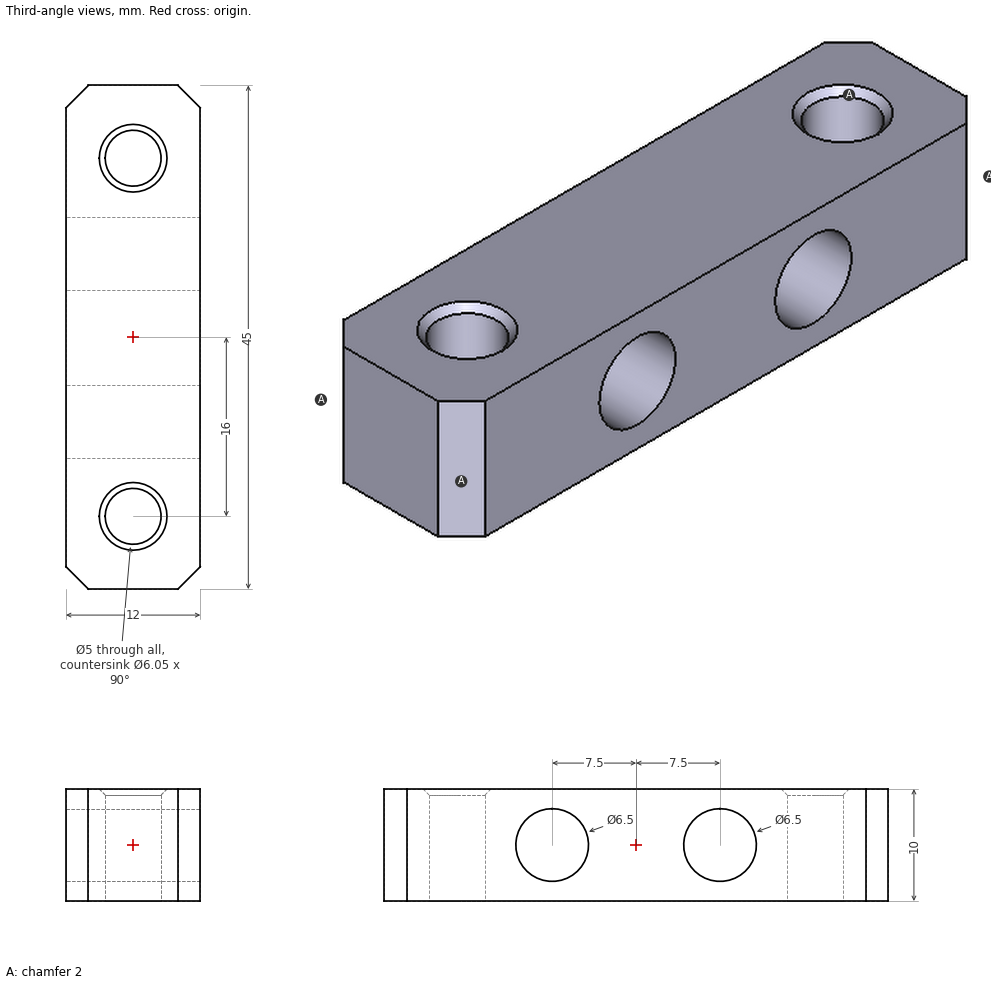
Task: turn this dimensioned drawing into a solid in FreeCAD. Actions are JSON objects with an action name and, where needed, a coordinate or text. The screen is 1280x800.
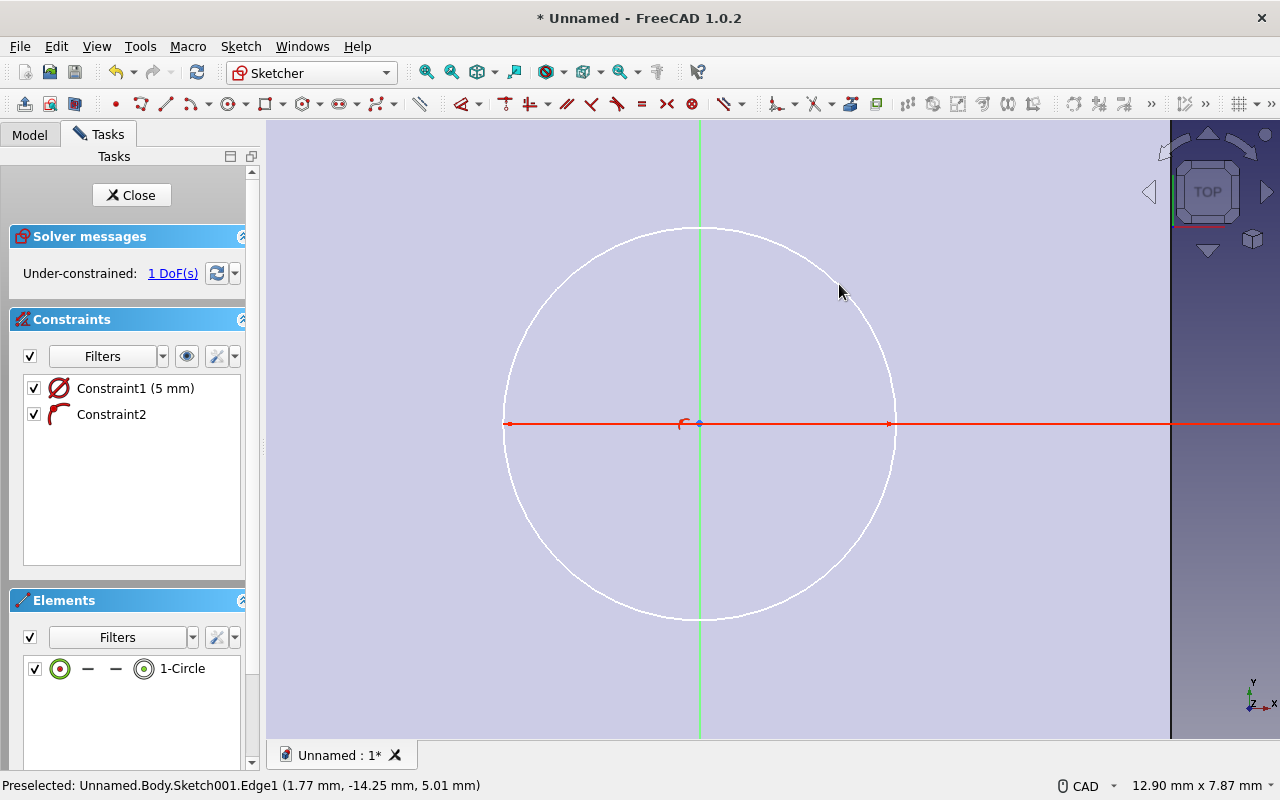
{"action": "left_click", "coordinate": [460, 104]}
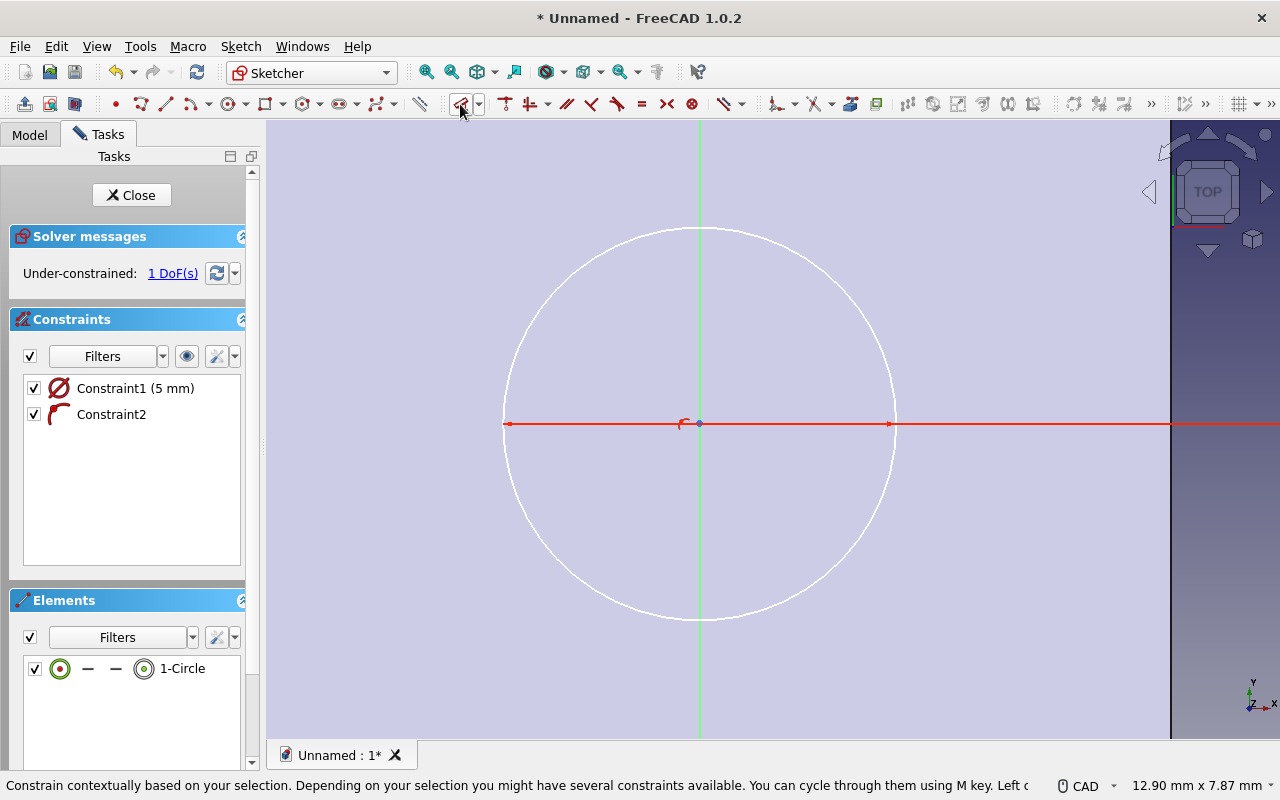
{"action": "left_click", "coordinate": [700, 424]}
{"action": "left_click", "coordinate": [734, 286]}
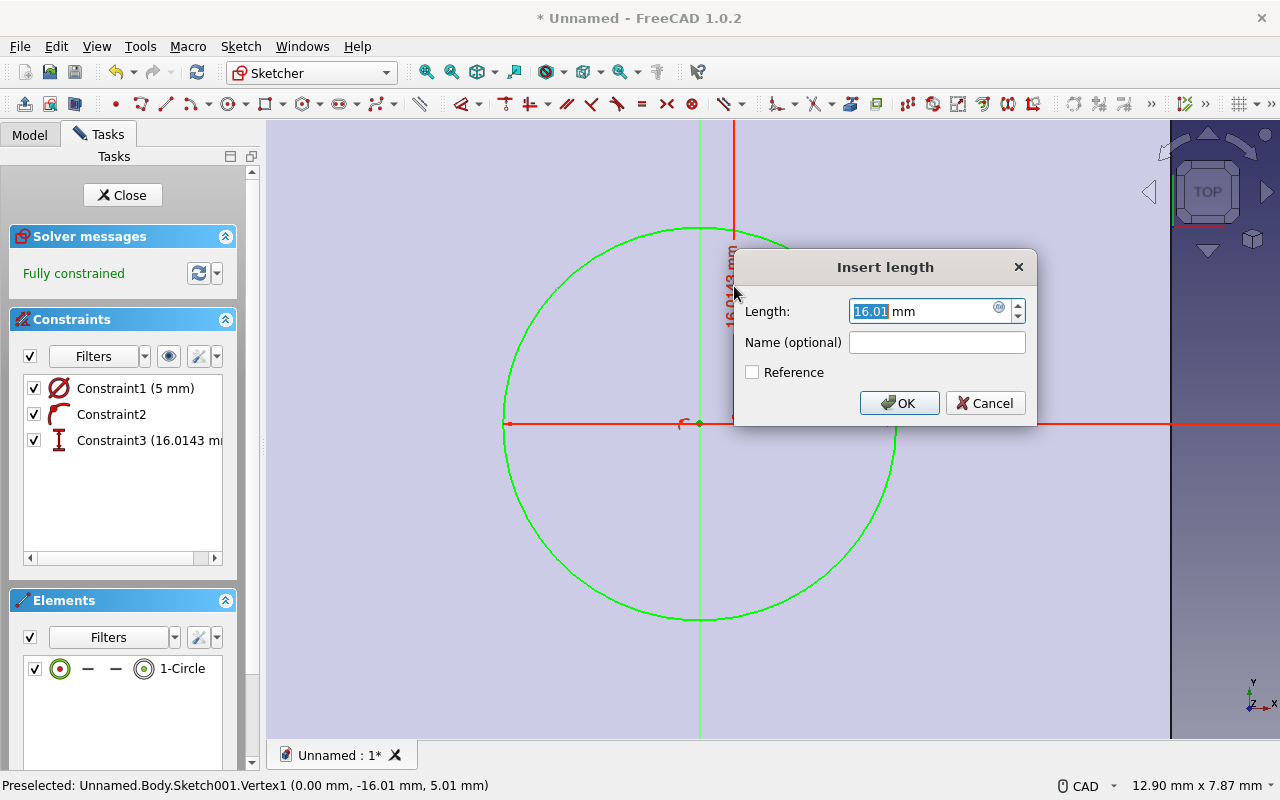
{"action": "type", "text": "16"}
{"action": "key", "text": "Return"}
{"action": "key", "text": "Escape"}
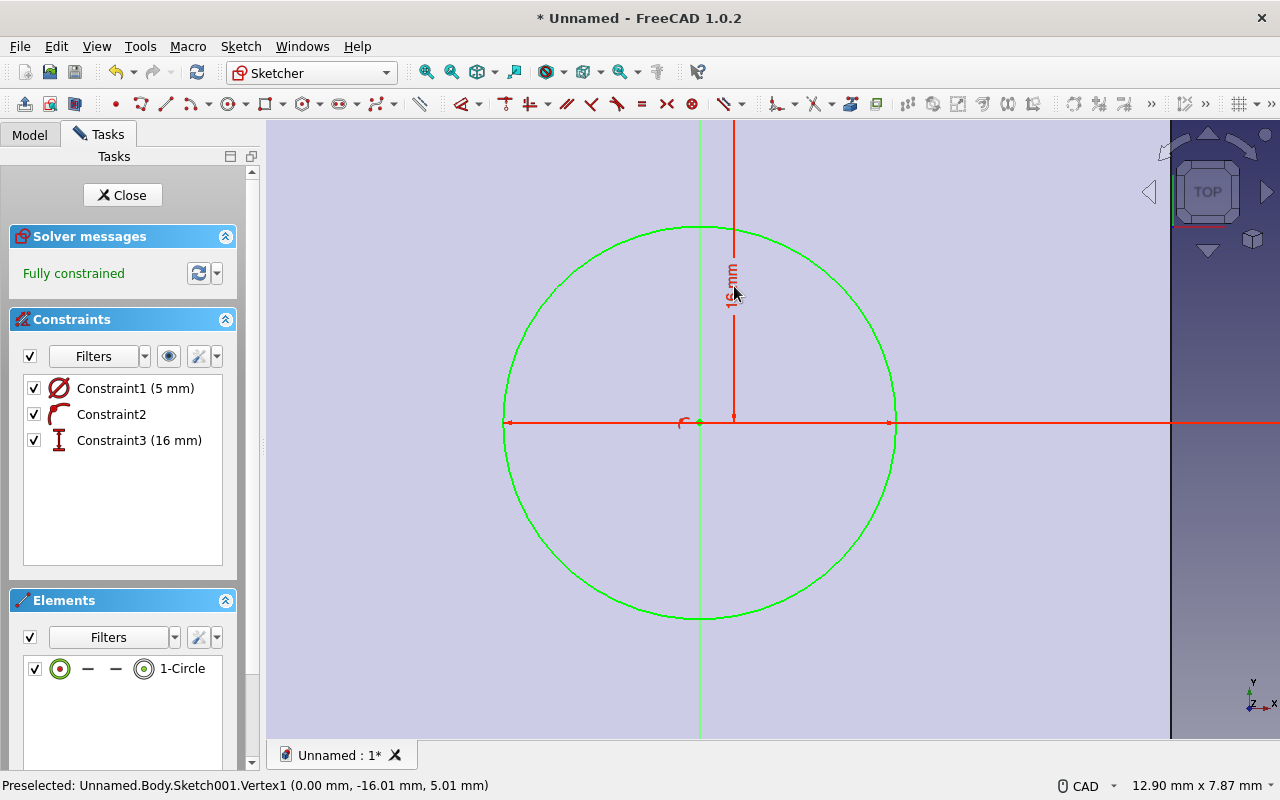
{"action": "left_click", "coordinate": [123, 195]}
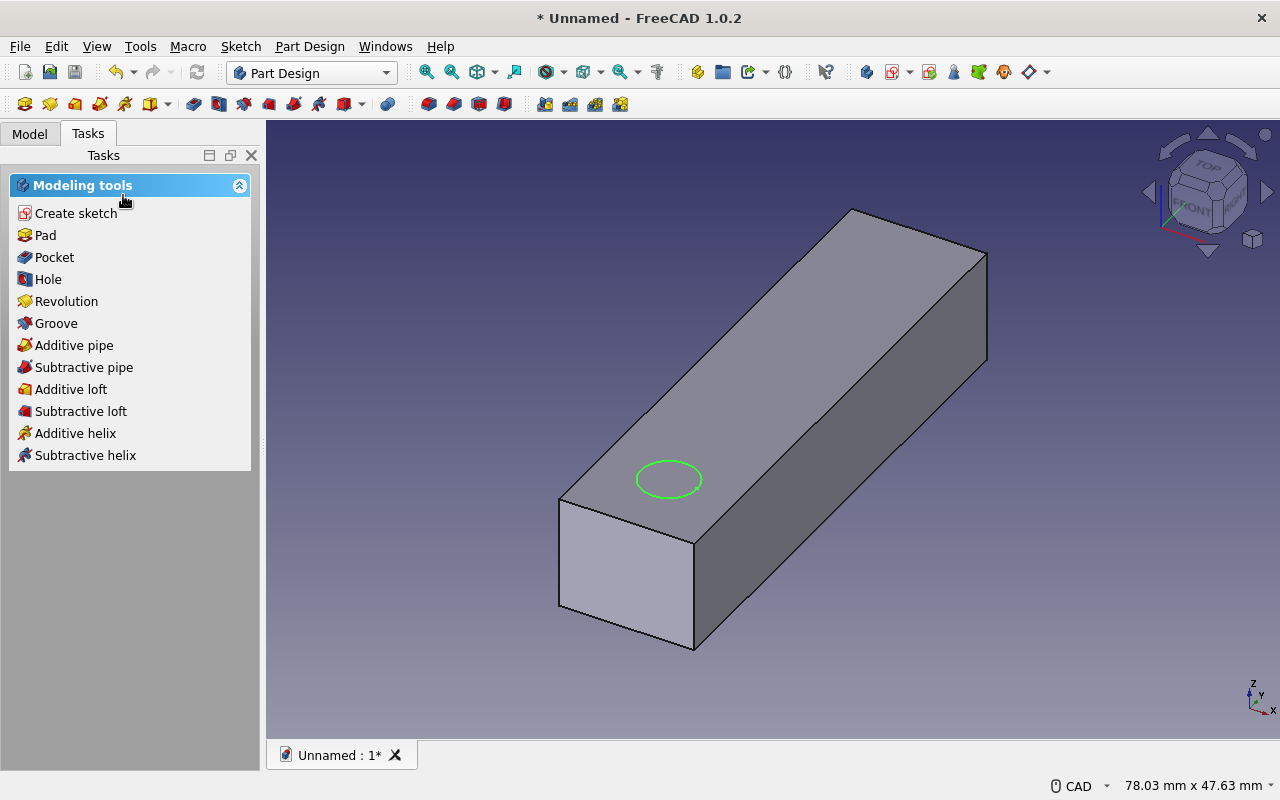
{"action": "left_click", "coordinate": [219, 104]}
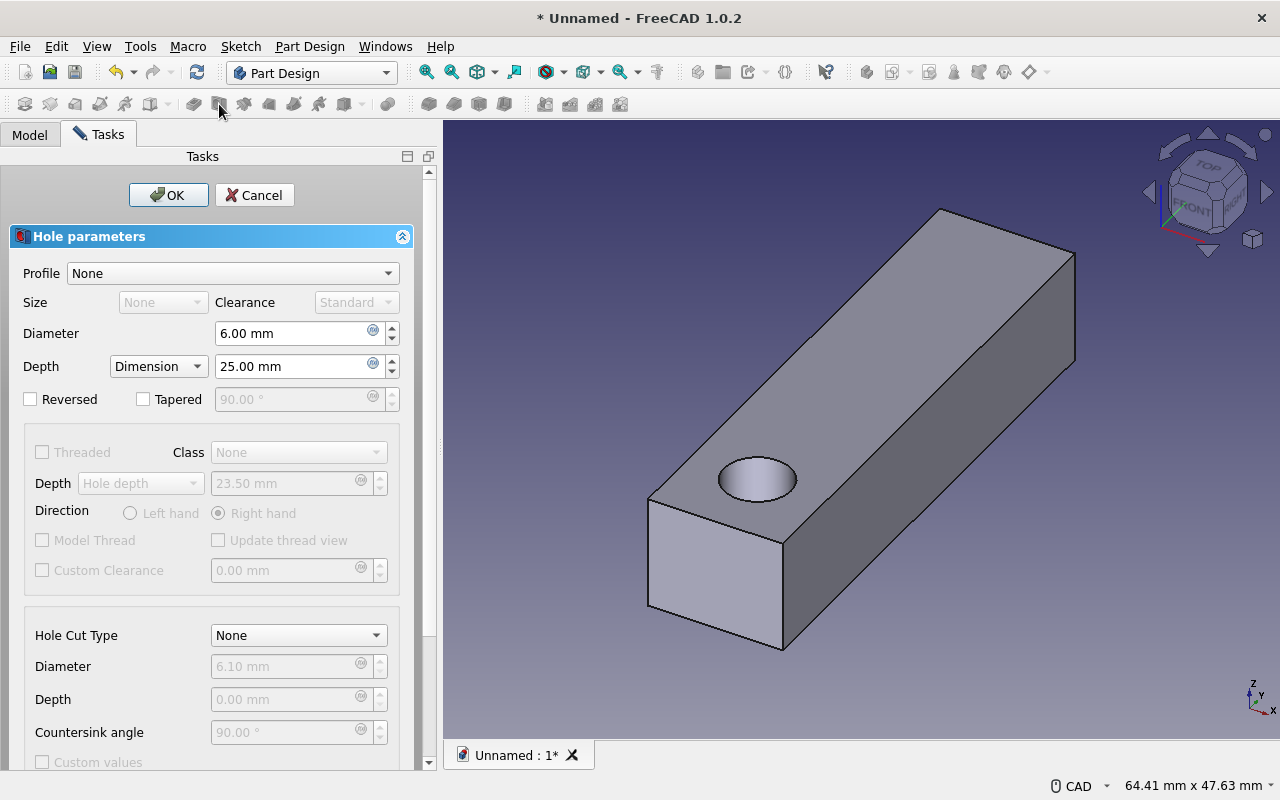
{"action": "triple_click", "coordinate": [300, 334]}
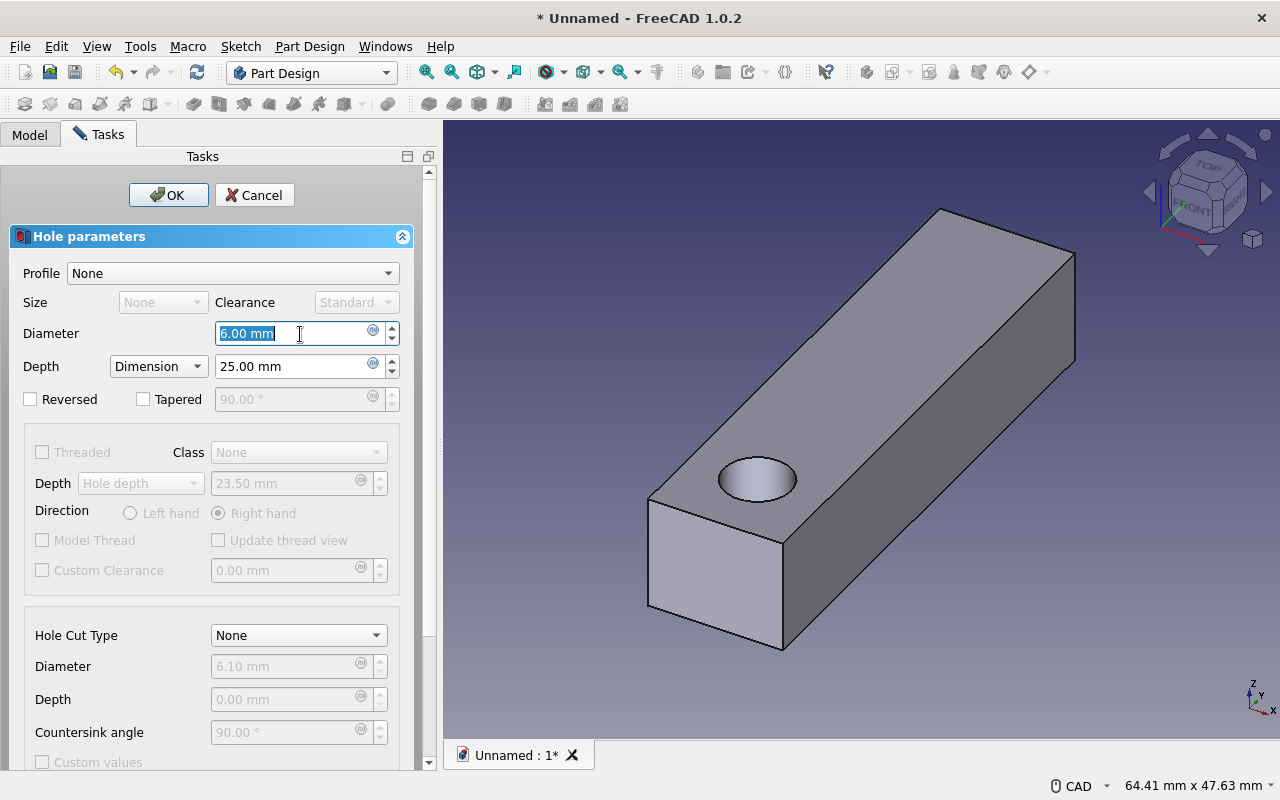
{"action": "type", "text": "5"}
{"action": "key", "text": "Tab"}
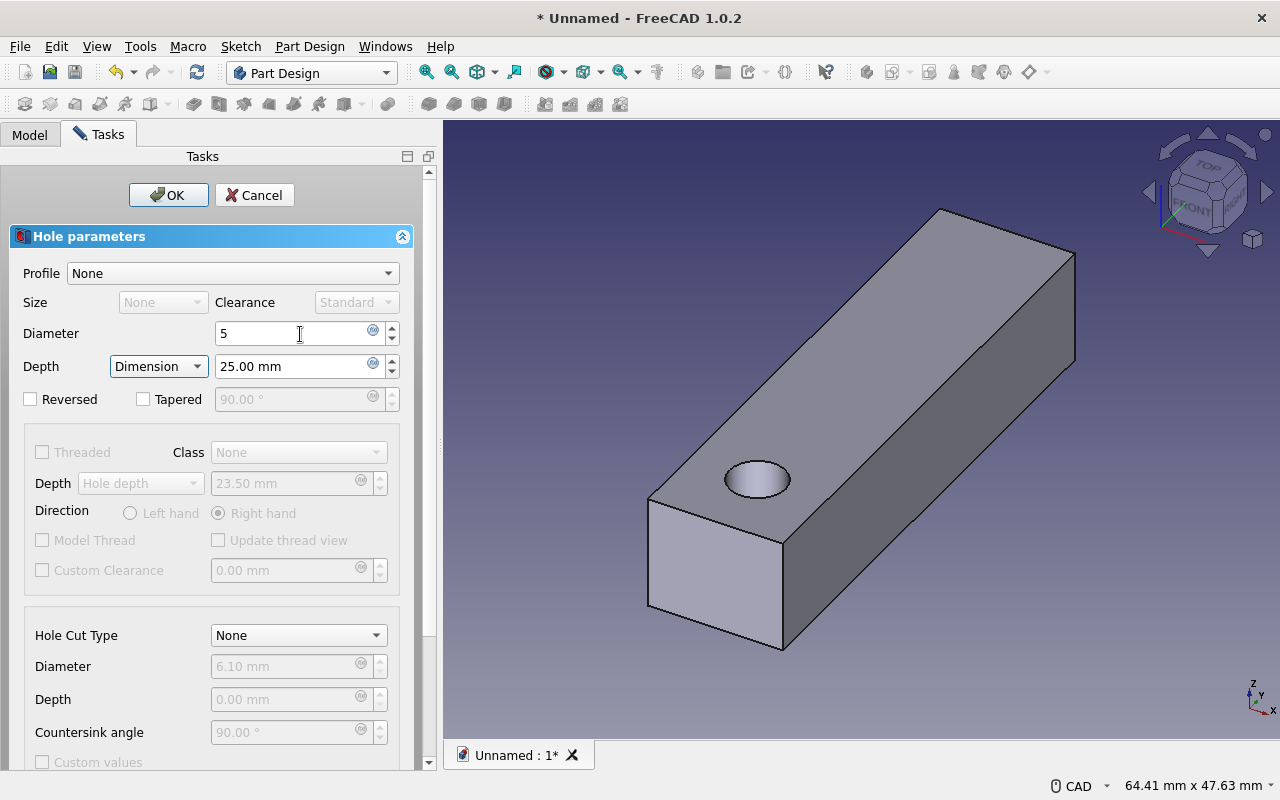
{"action": "left_click", "coordinate": [160, 366]}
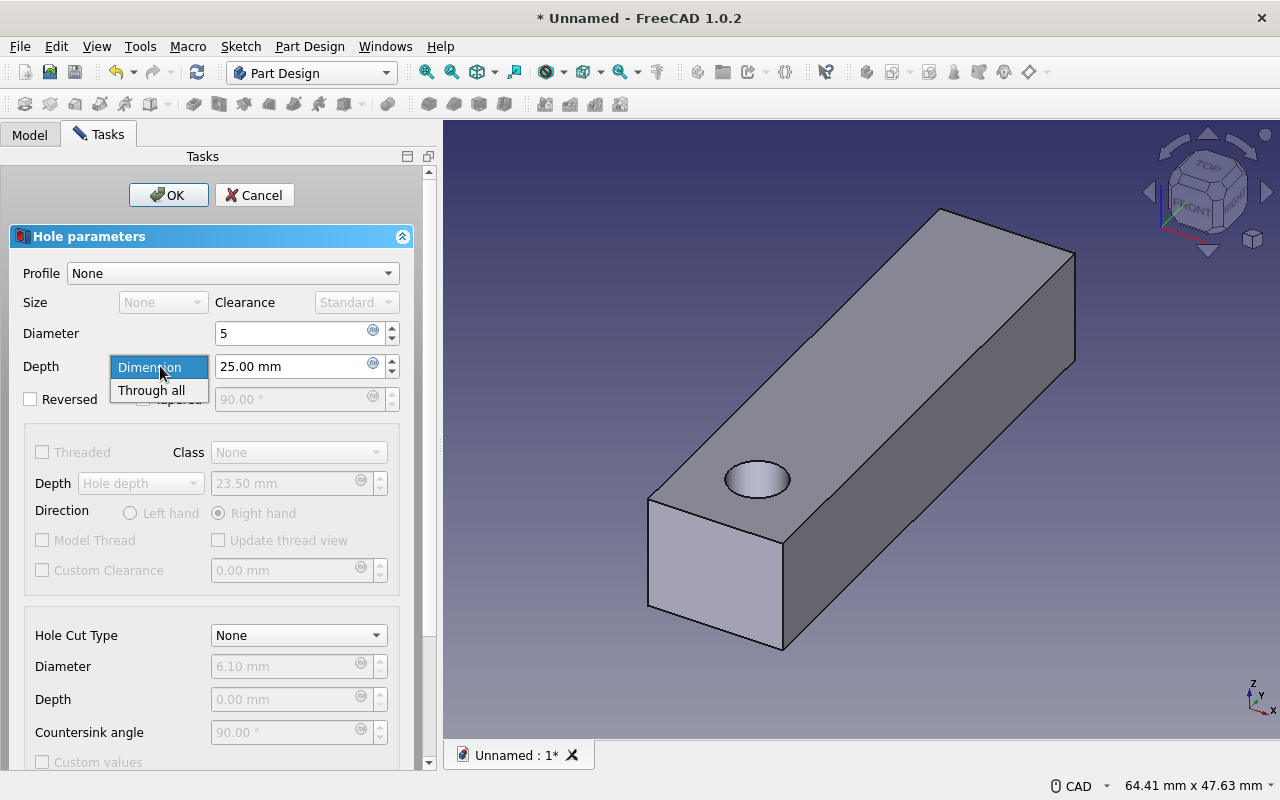
{"action": "left_click", "coordinate": [158, 390]}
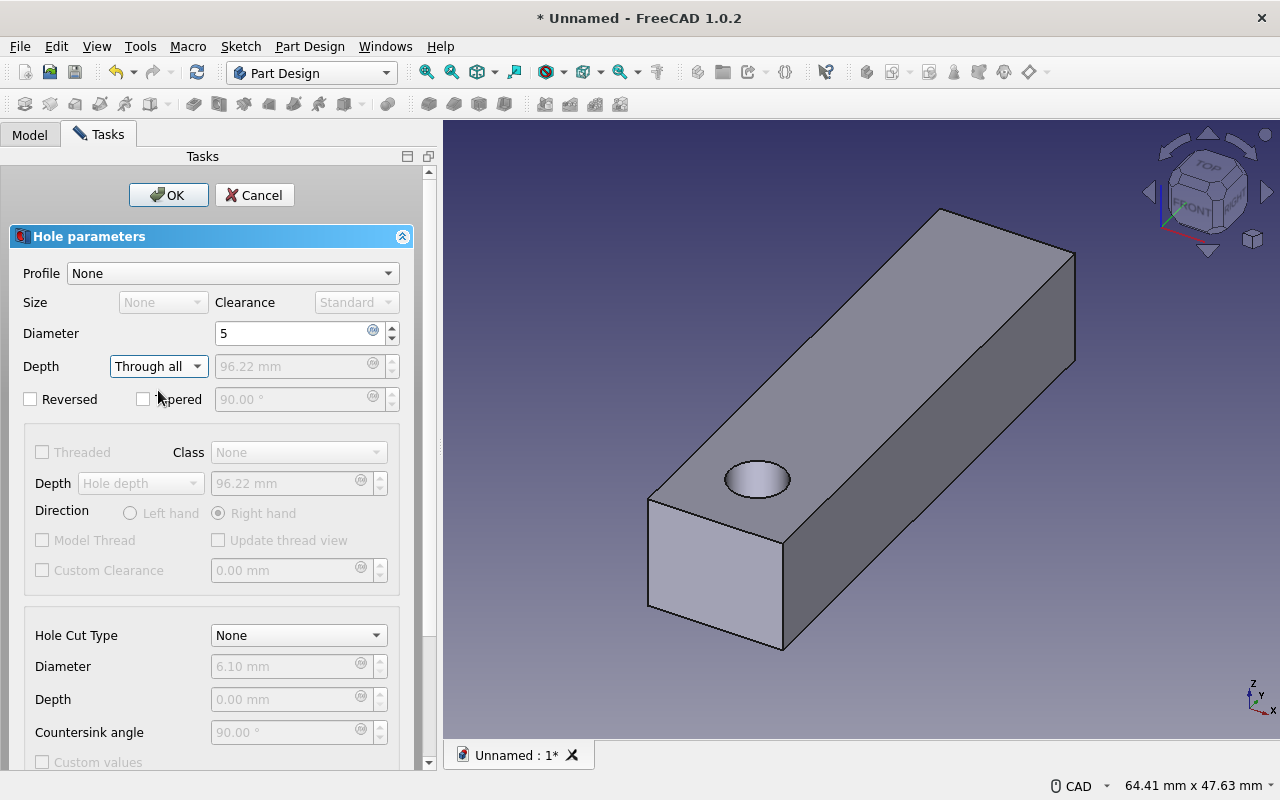
{"action": "left_click", "coordinate": [300, 636]}